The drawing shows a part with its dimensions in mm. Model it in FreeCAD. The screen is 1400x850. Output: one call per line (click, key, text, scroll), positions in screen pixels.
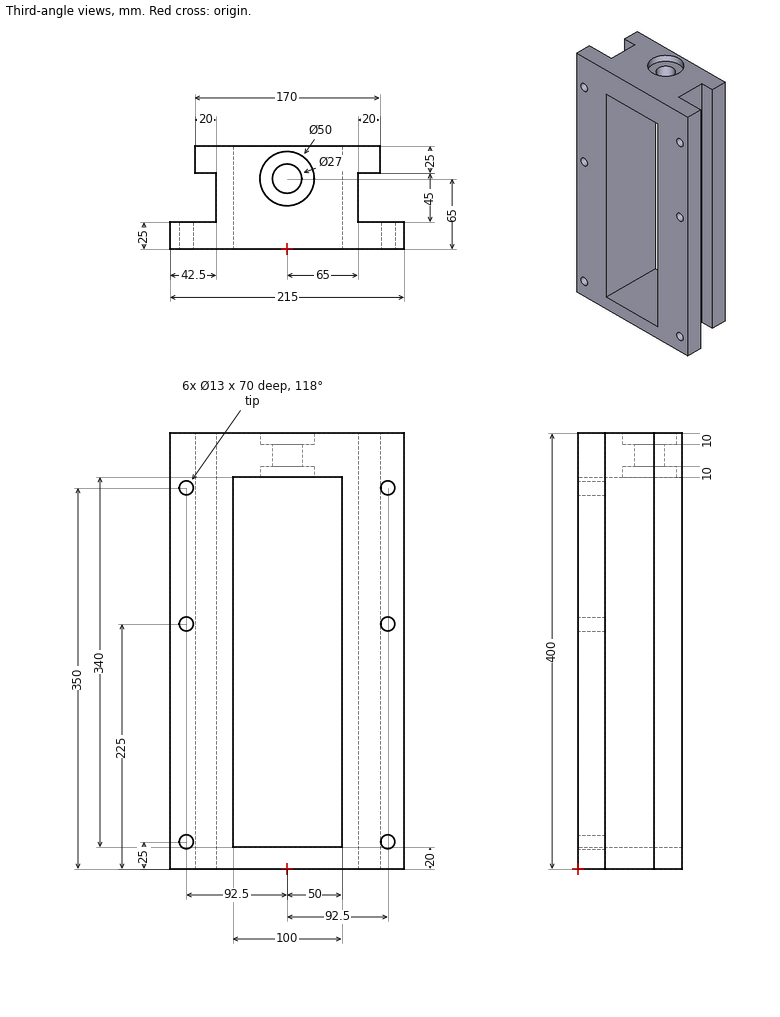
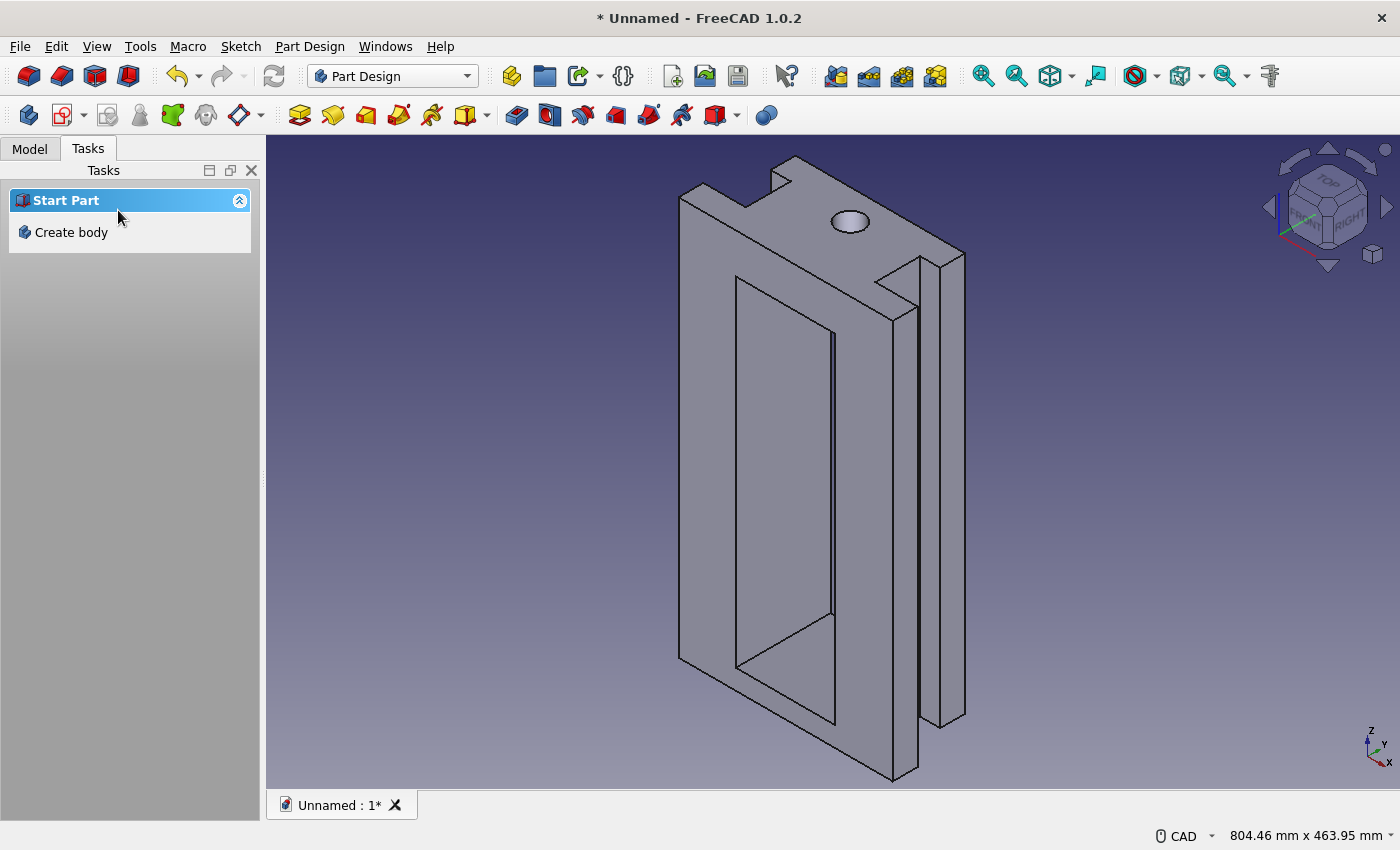
click(850, 256)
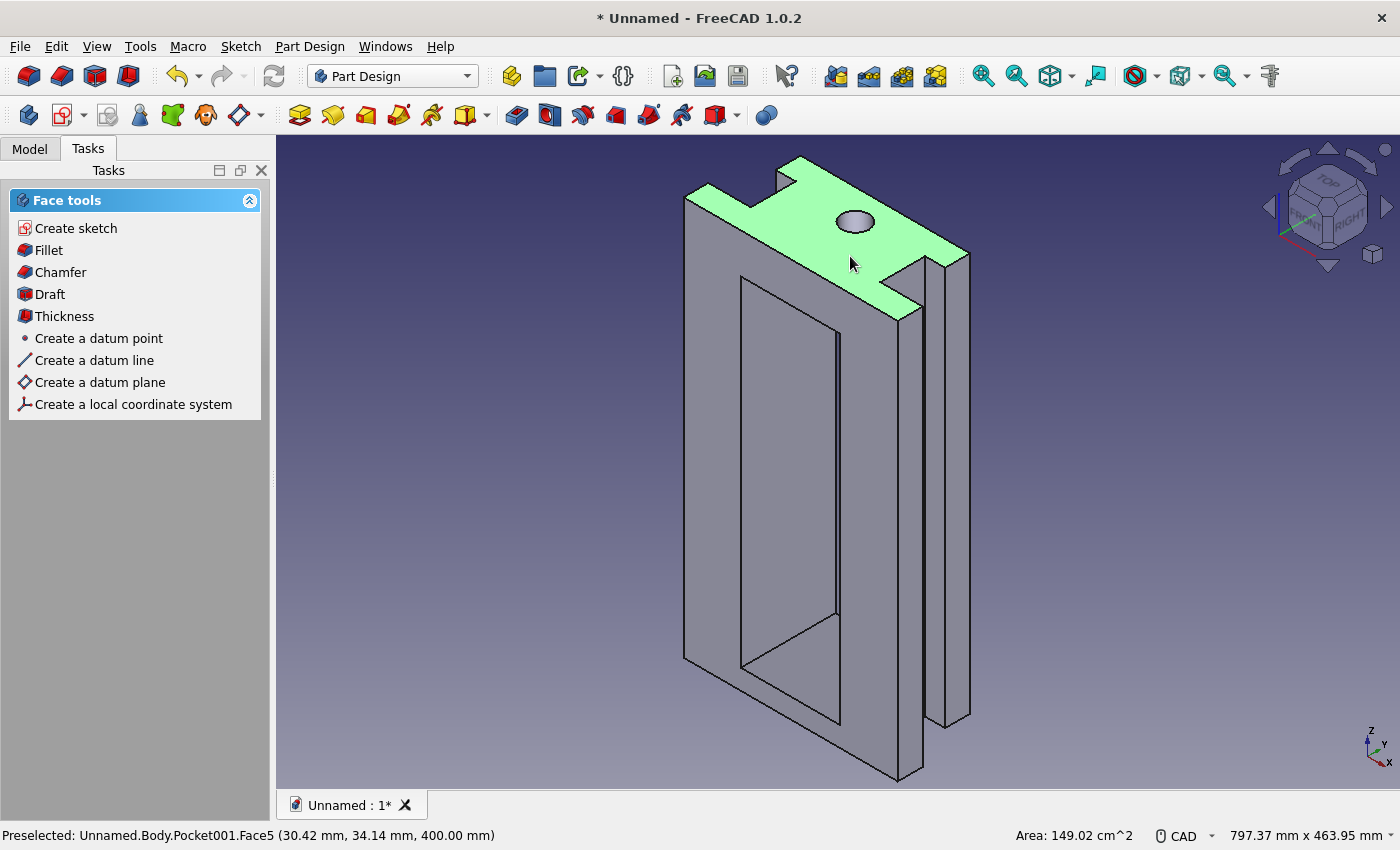
click(62, 116)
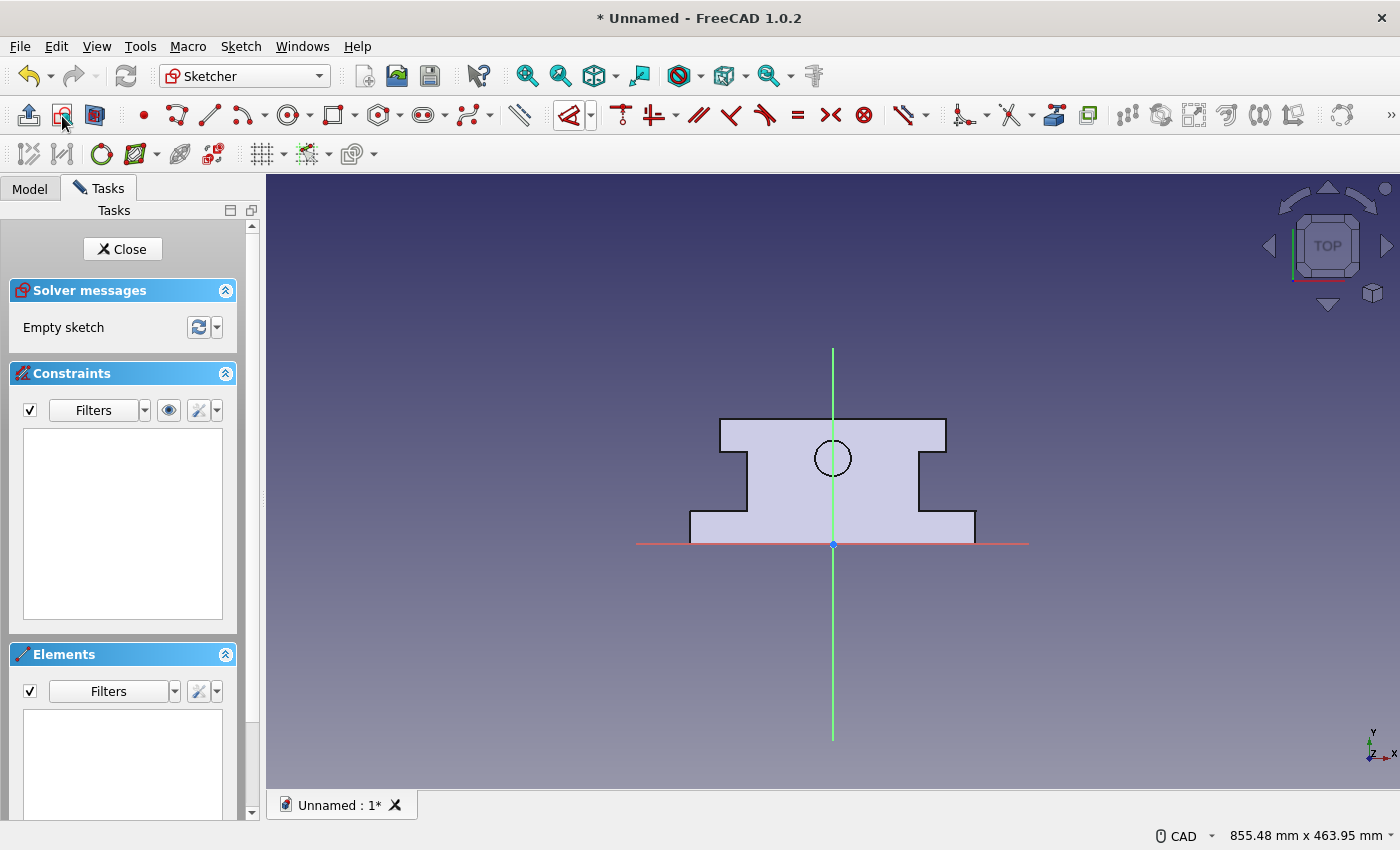
scroll(863, 486, up, 6)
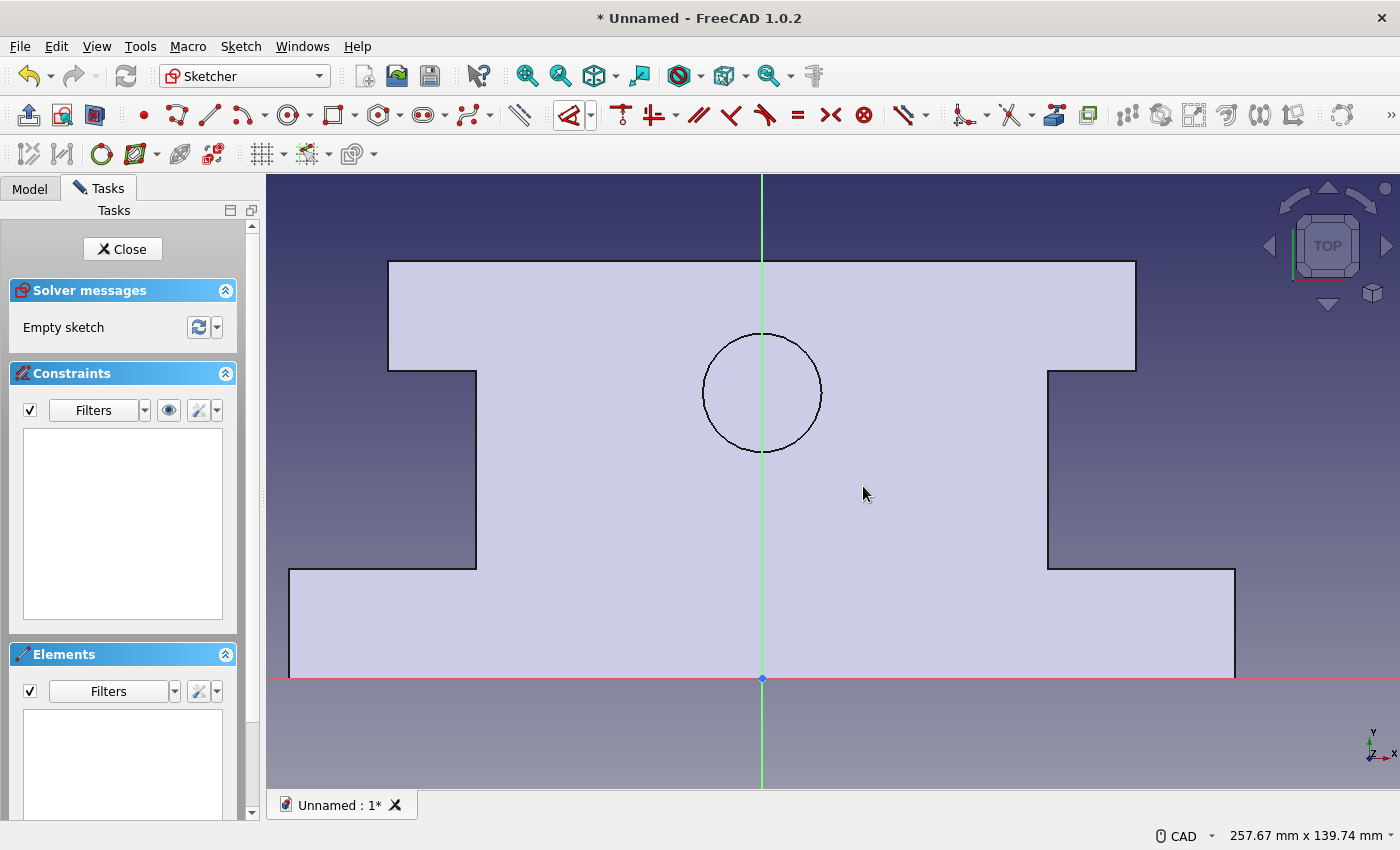
key(g)
key(c)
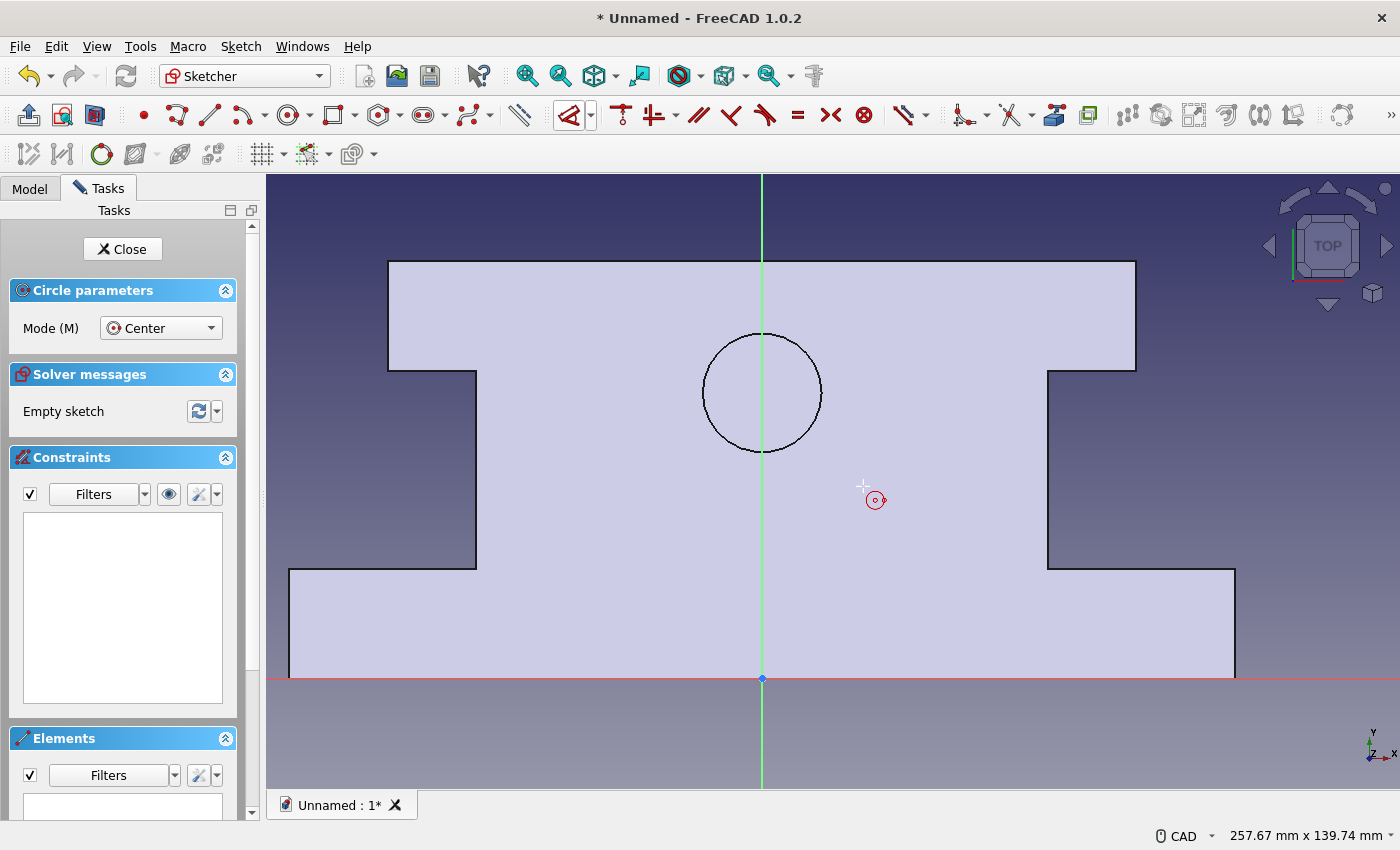
click(762, 393)
move(840, 315)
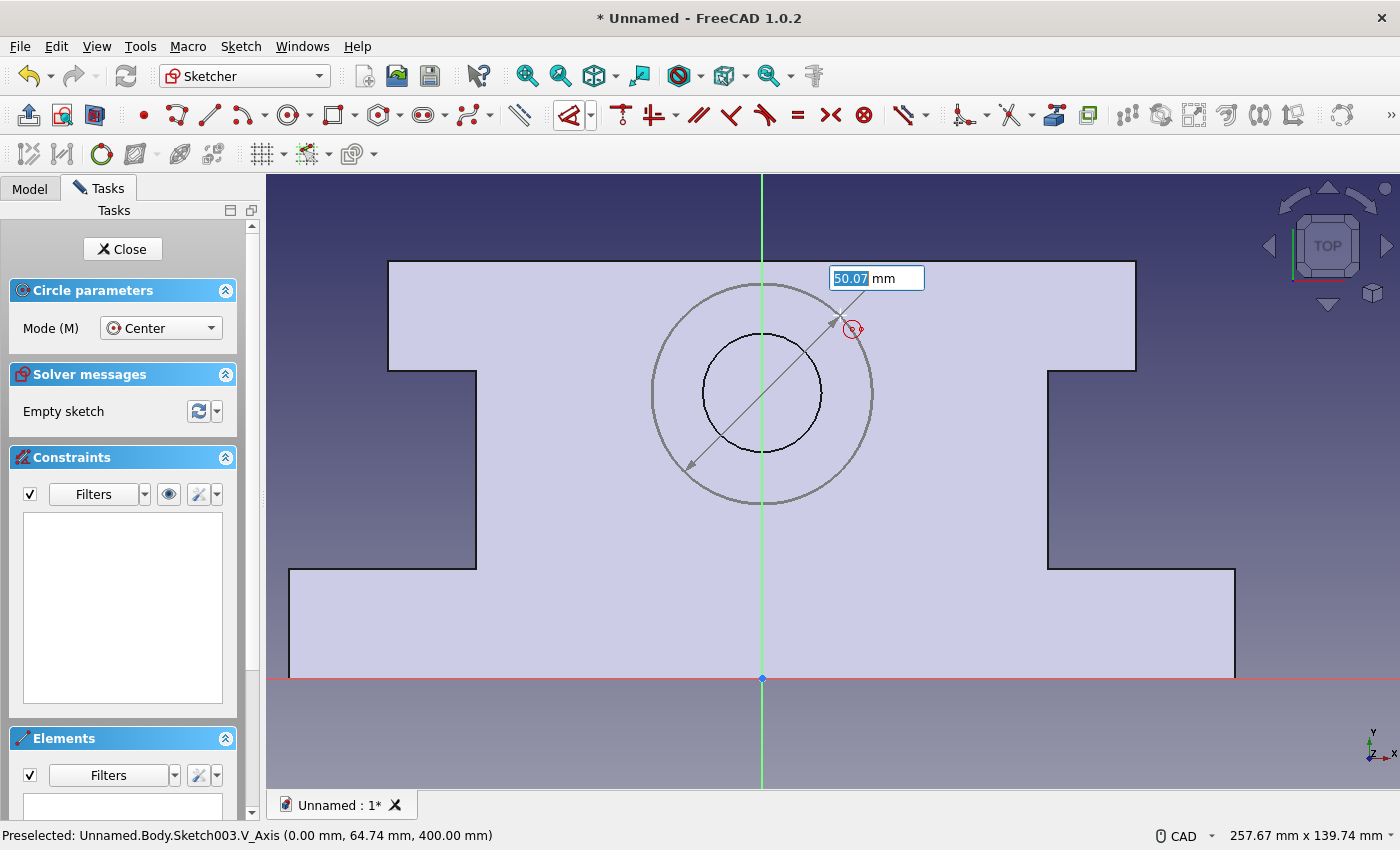
text(50)
key(Return)
key(Escape)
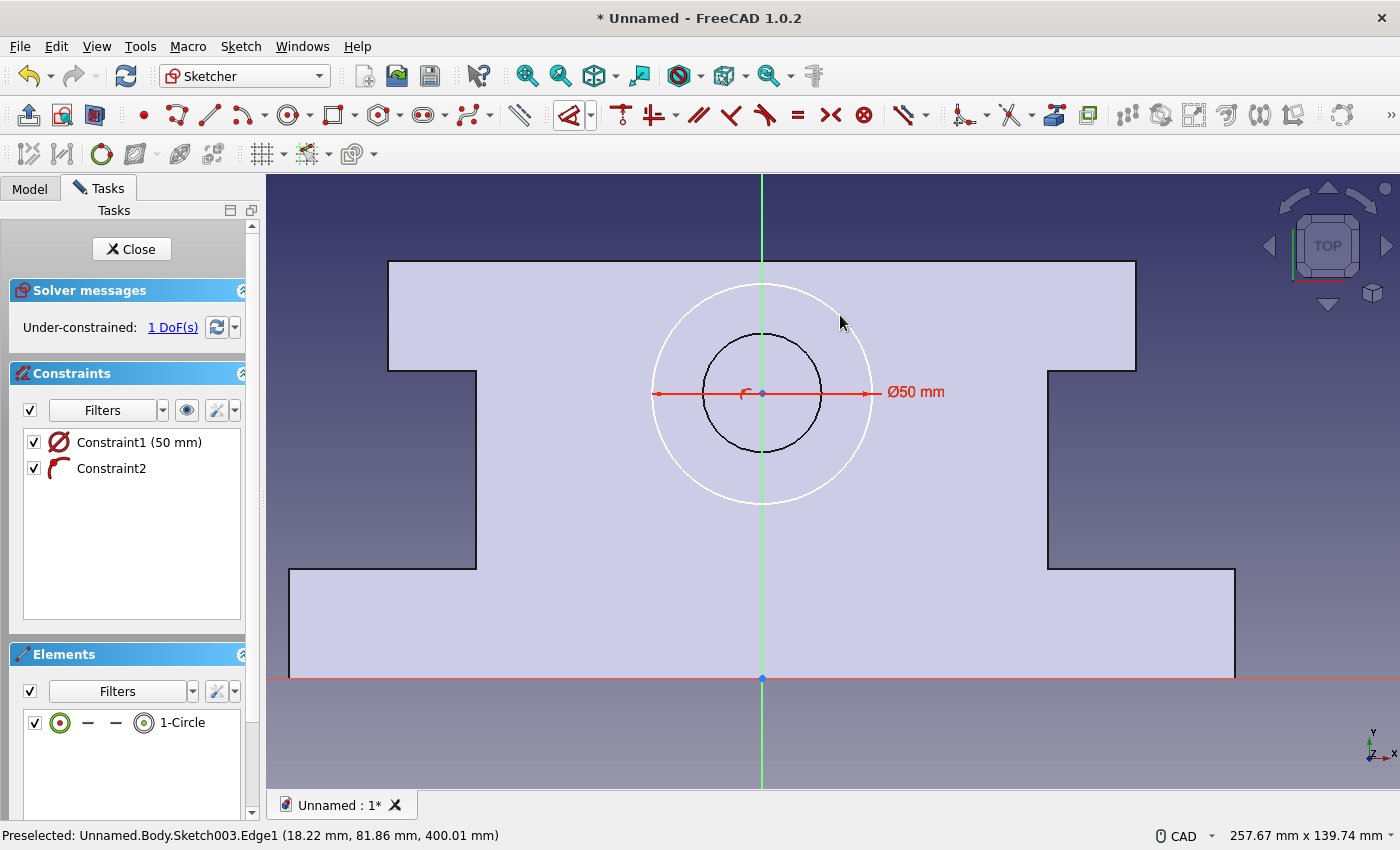
click(762, 394)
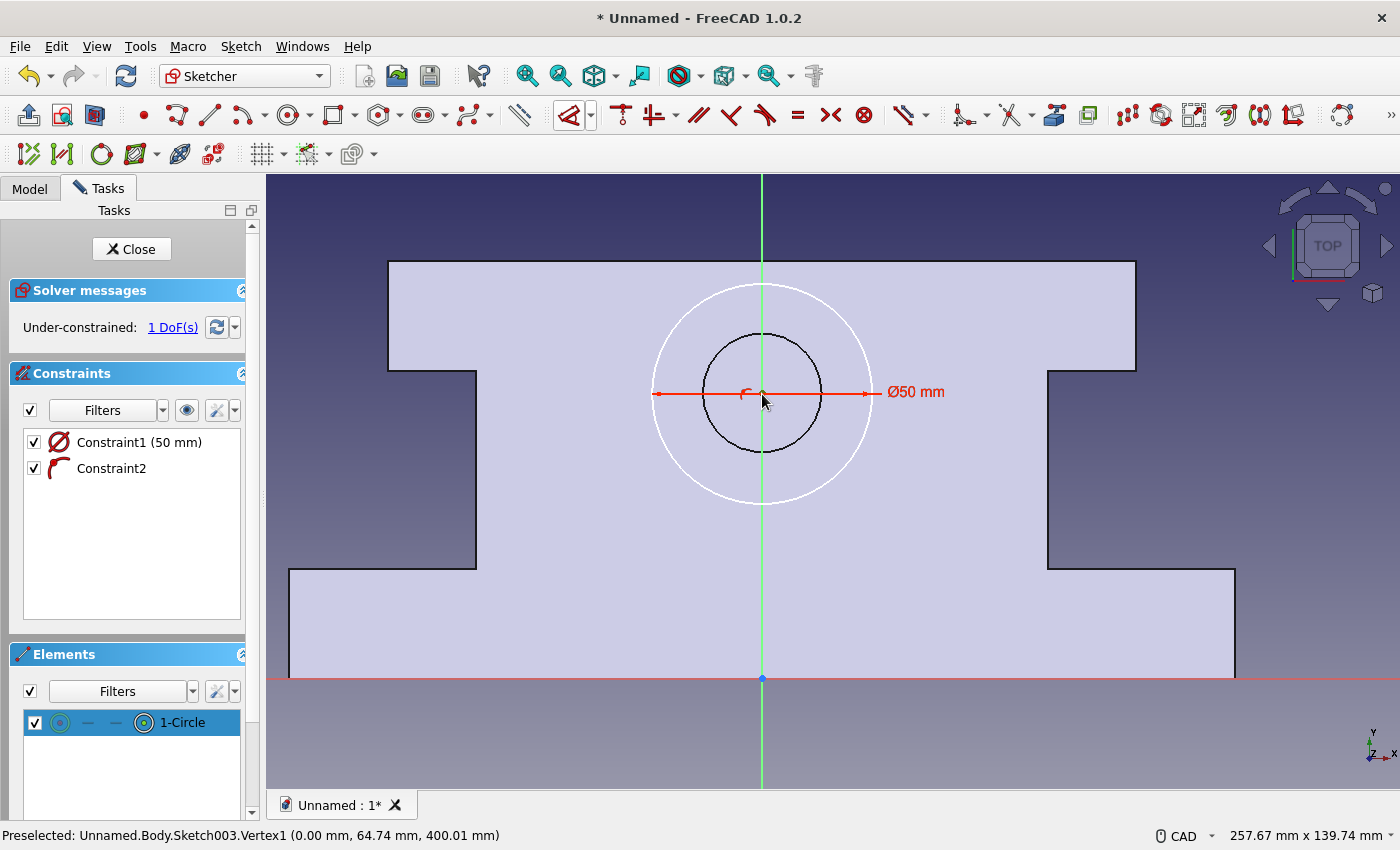
key(i)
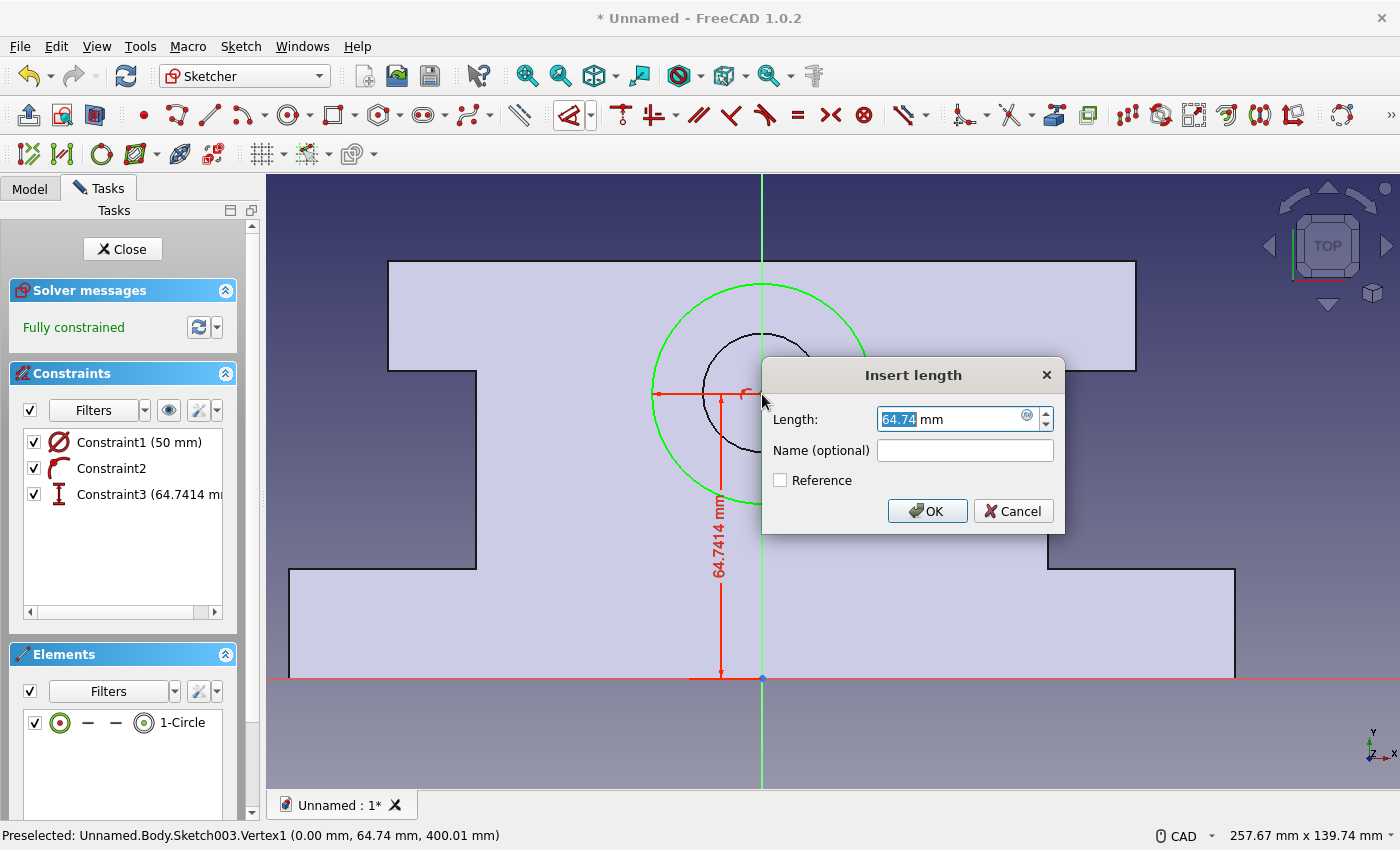
text(65)
key(Return)